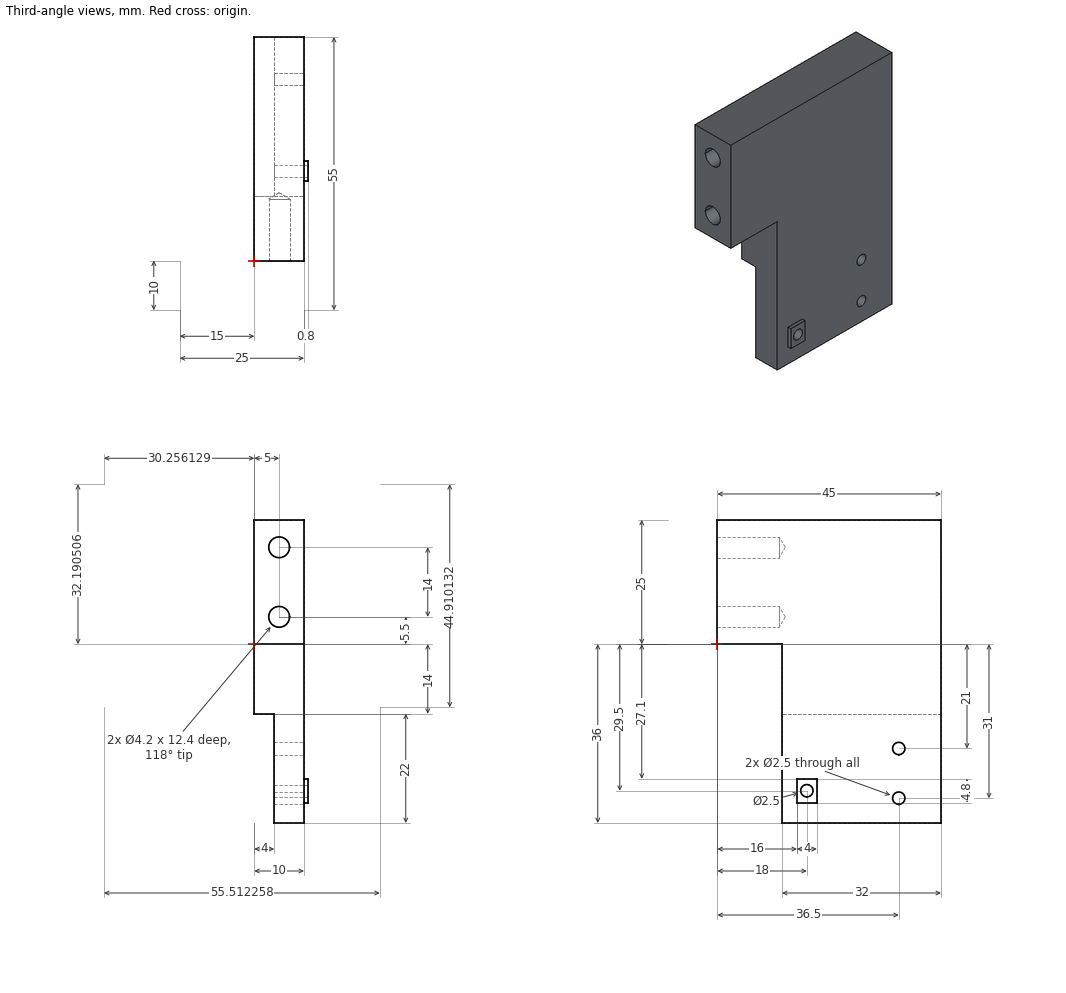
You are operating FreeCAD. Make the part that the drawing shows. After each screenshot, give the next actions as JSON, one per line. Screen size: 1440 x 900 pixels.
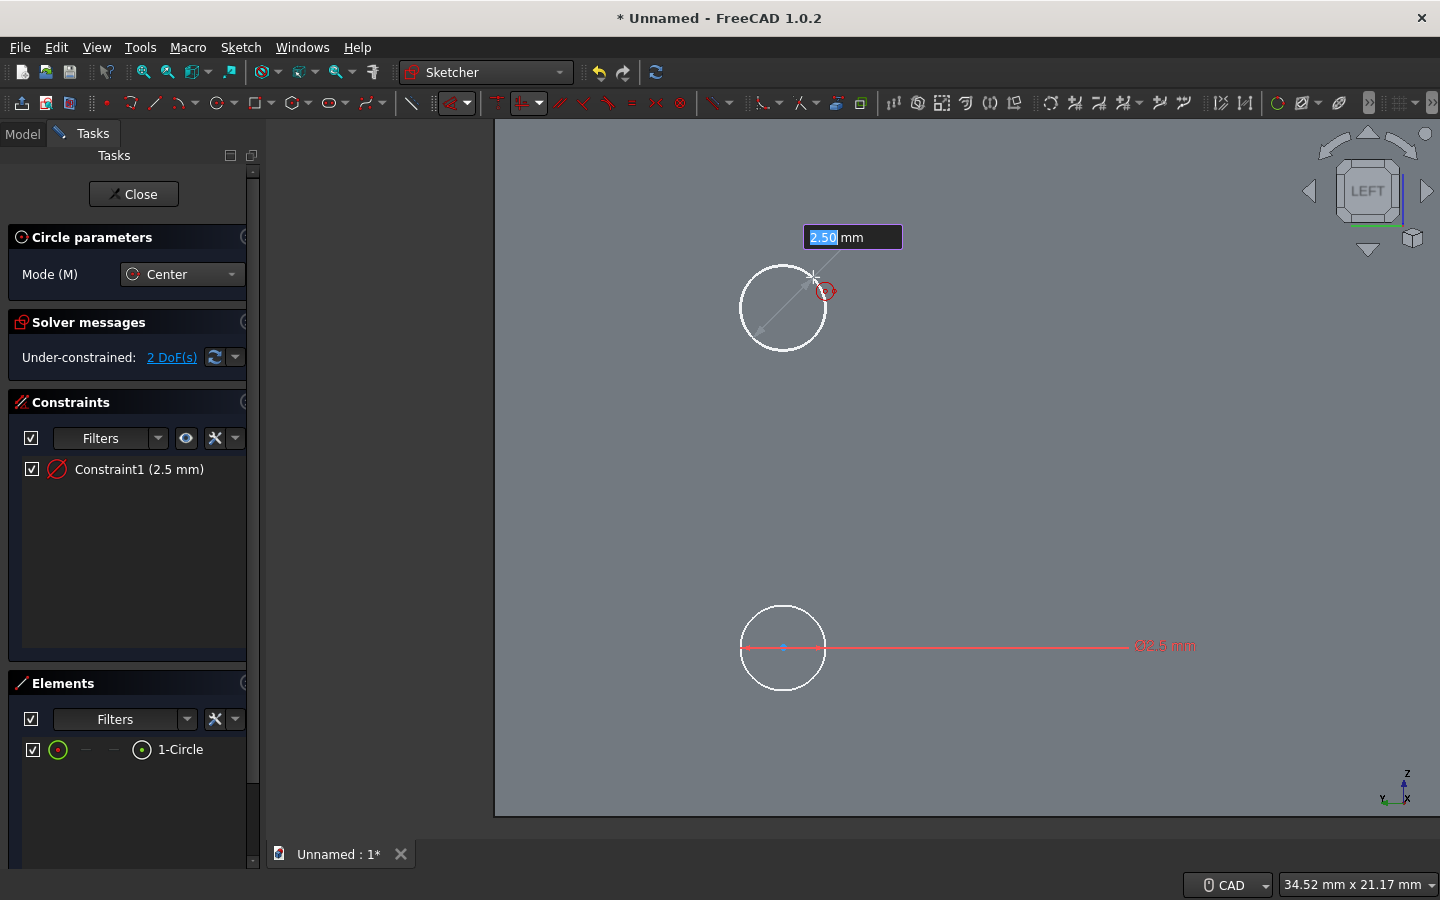
{"action": "type", "text": "2.5"}
{"action": "key", "text": "Return"}
{"action": "key", "text": "Escape"}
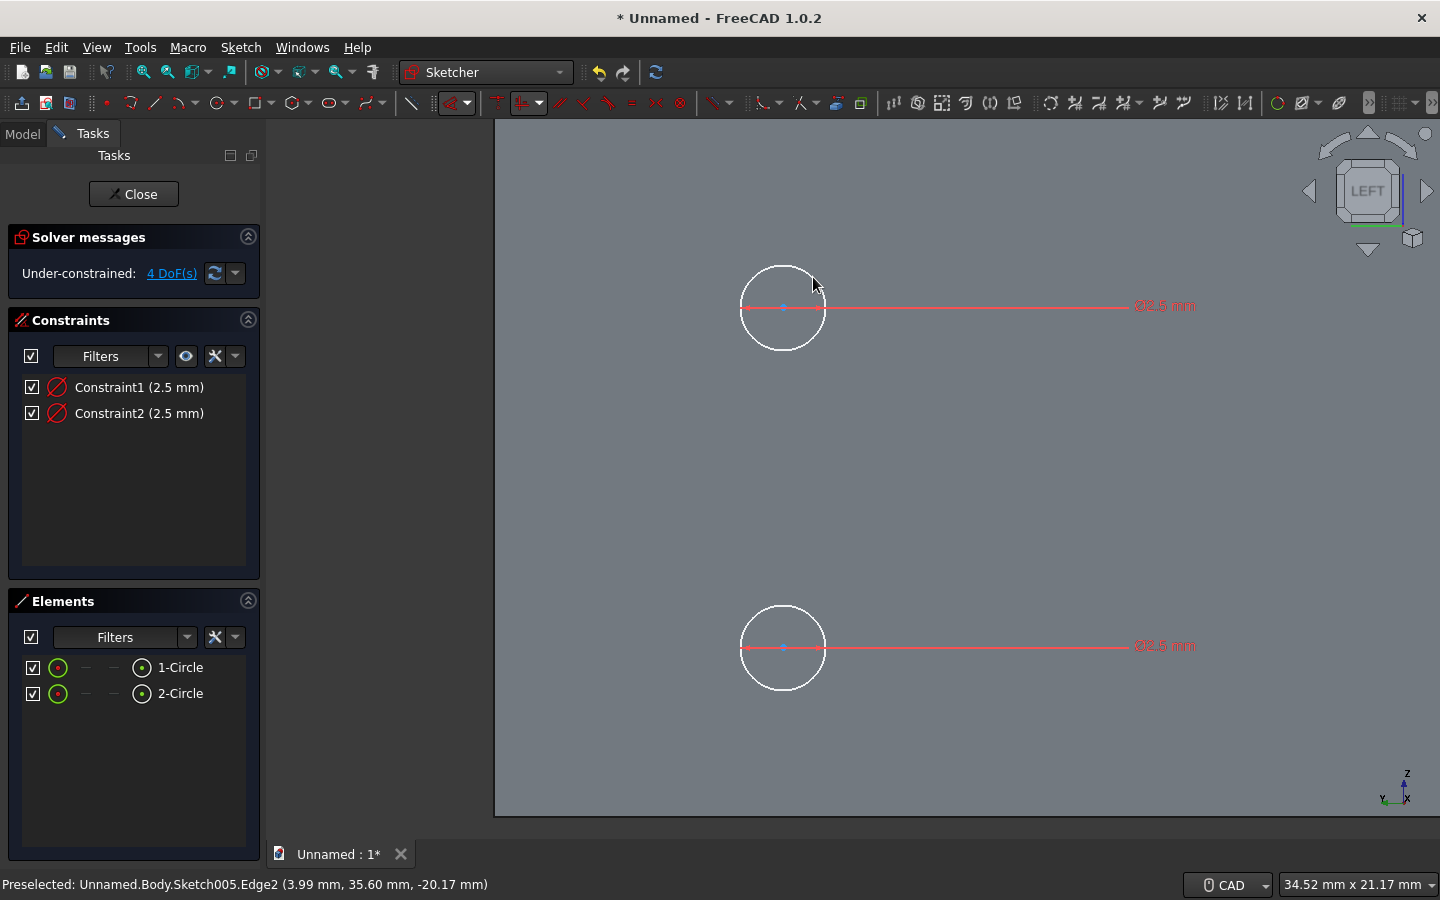
{"action": "left_click", "coordinate": [783, 648]}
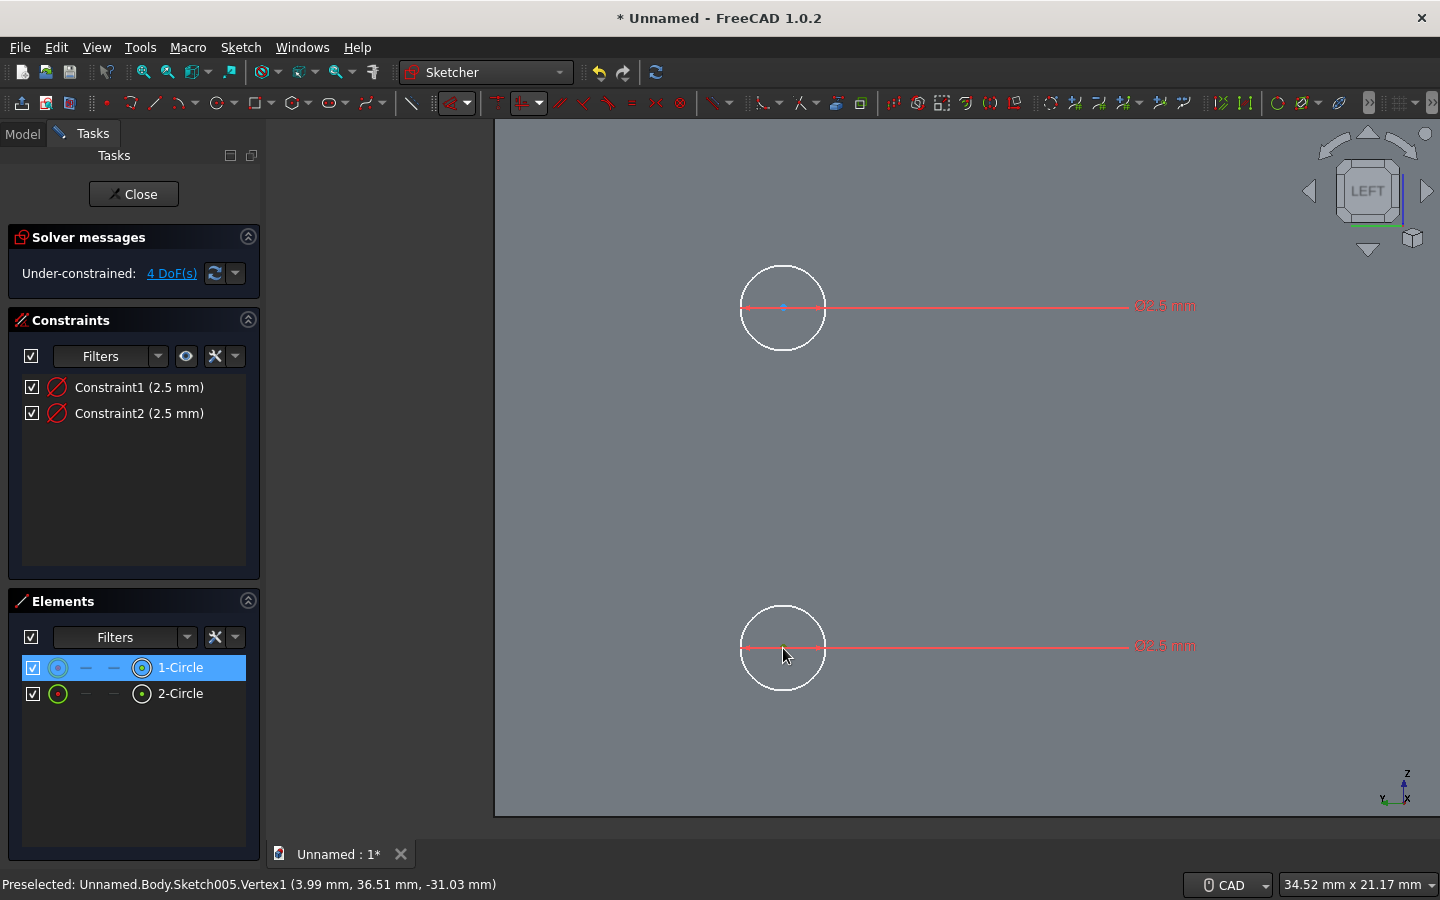
{"action": "left_click", "coordinate": [783, 308]}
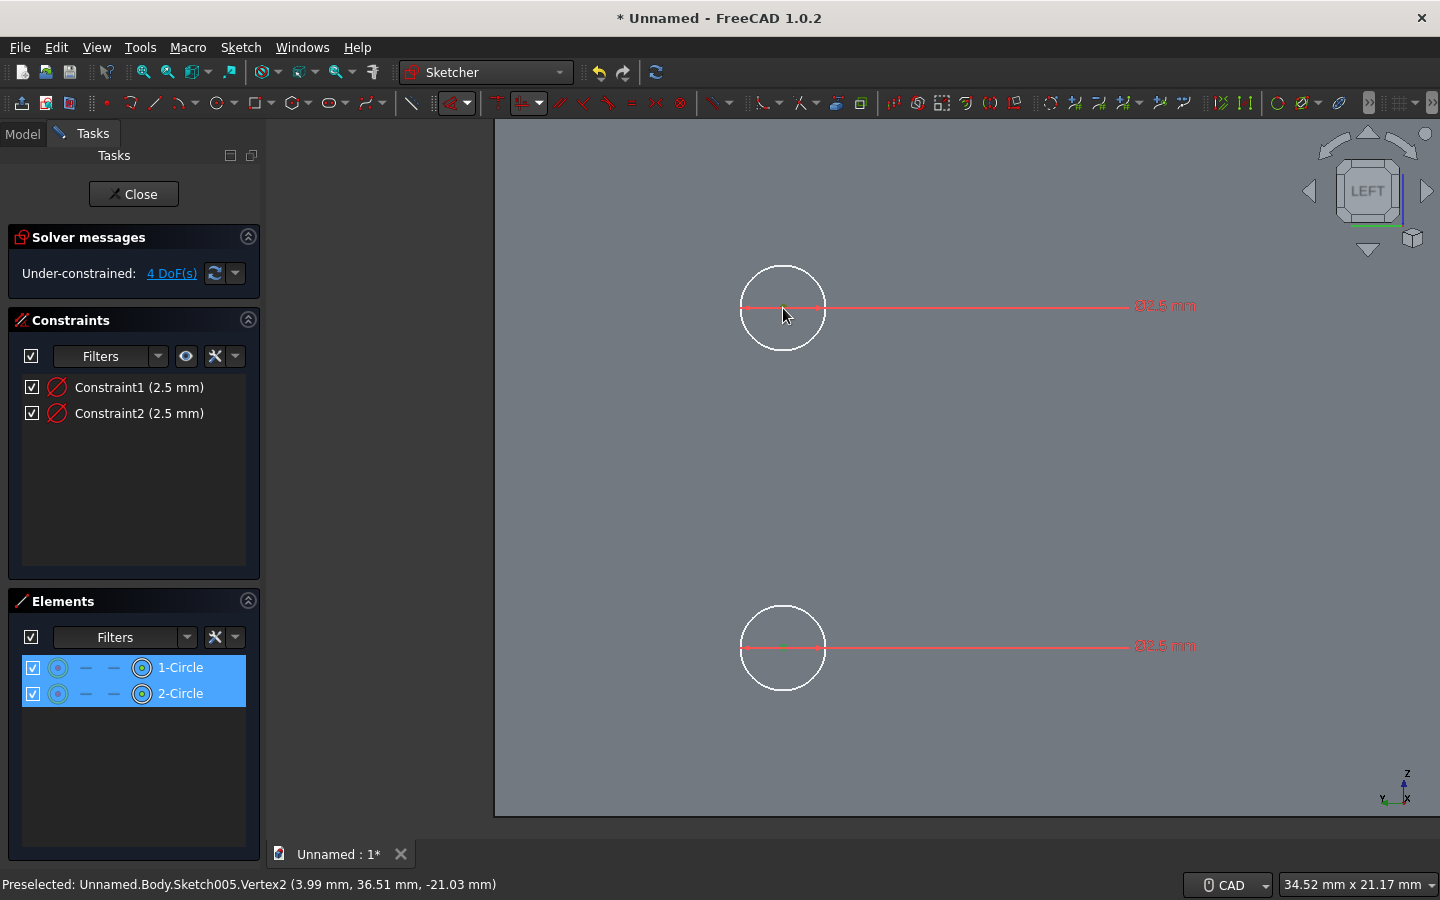
{"action": "left_click", "coordinate": [542, 104]}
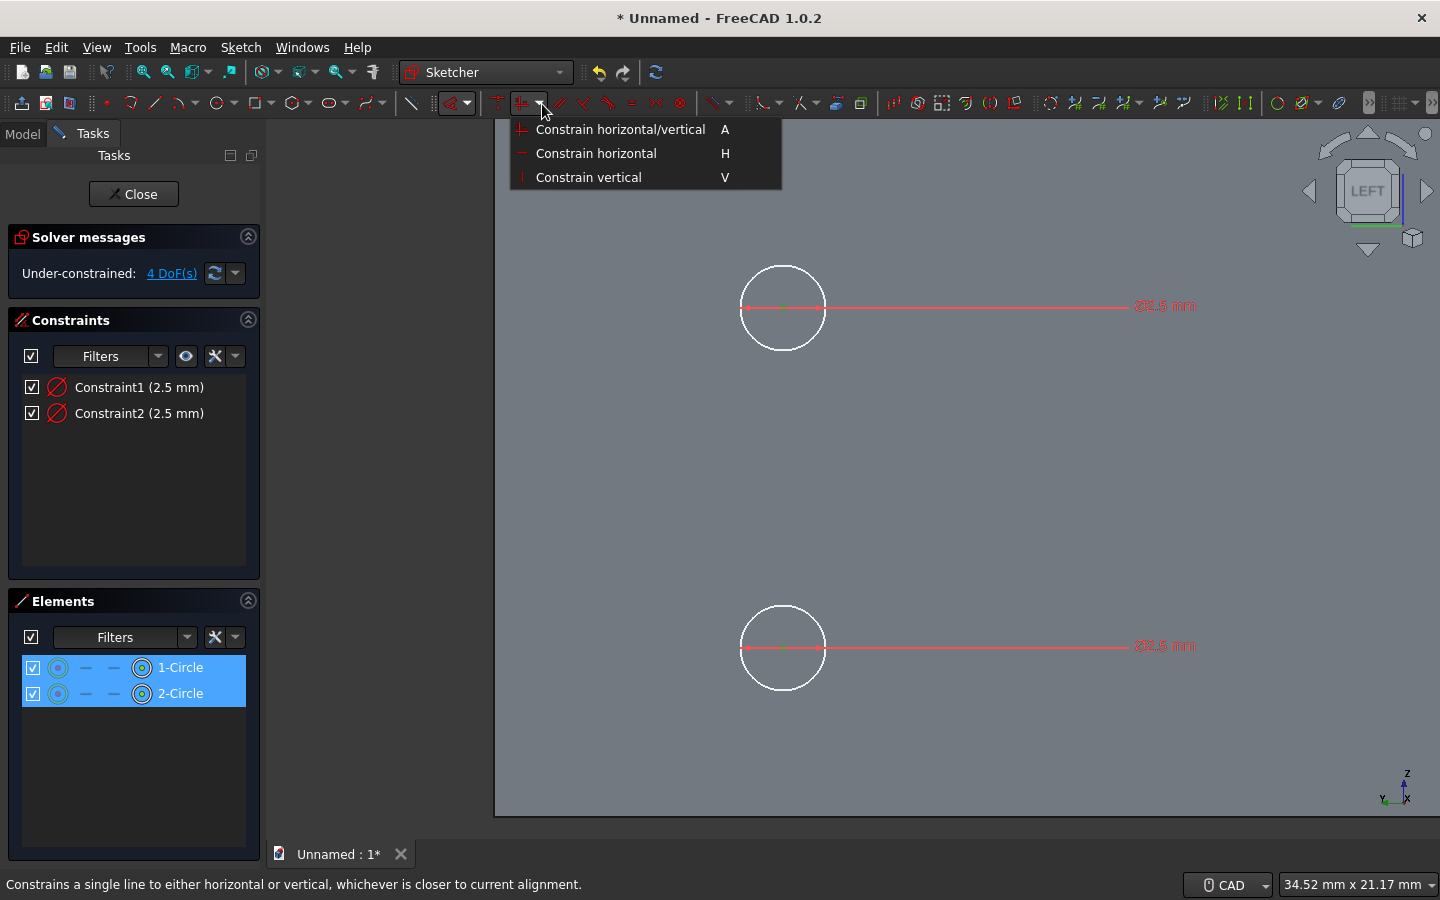
{"action": "left_click", "coordinate": [646, 177]}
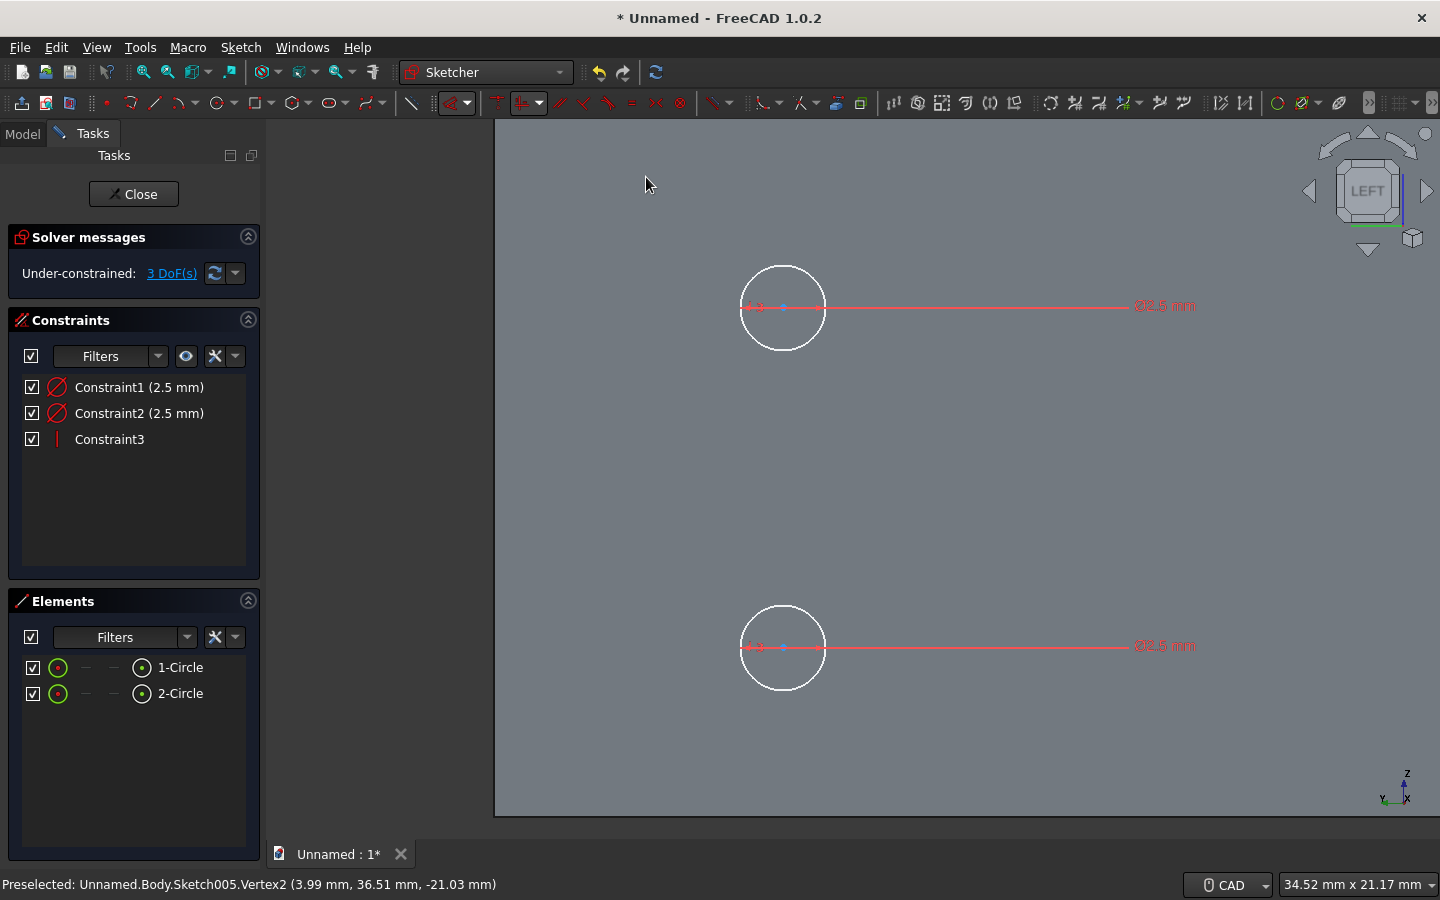
{"action": "left_click", "coordinate": [783, 648]}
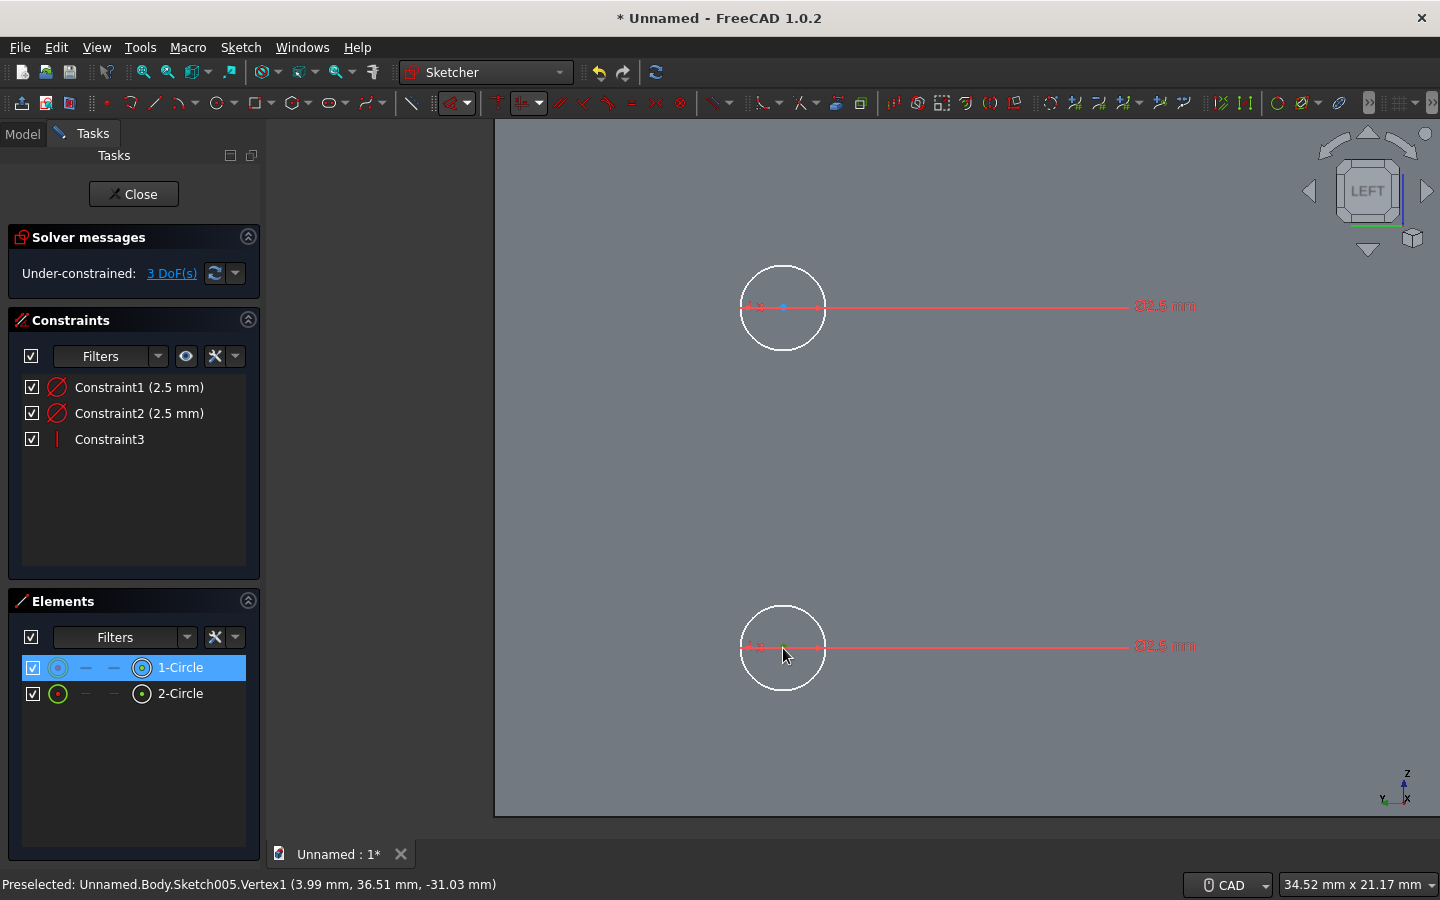
{"action": "left_click", "coordinate": [470, 104]}